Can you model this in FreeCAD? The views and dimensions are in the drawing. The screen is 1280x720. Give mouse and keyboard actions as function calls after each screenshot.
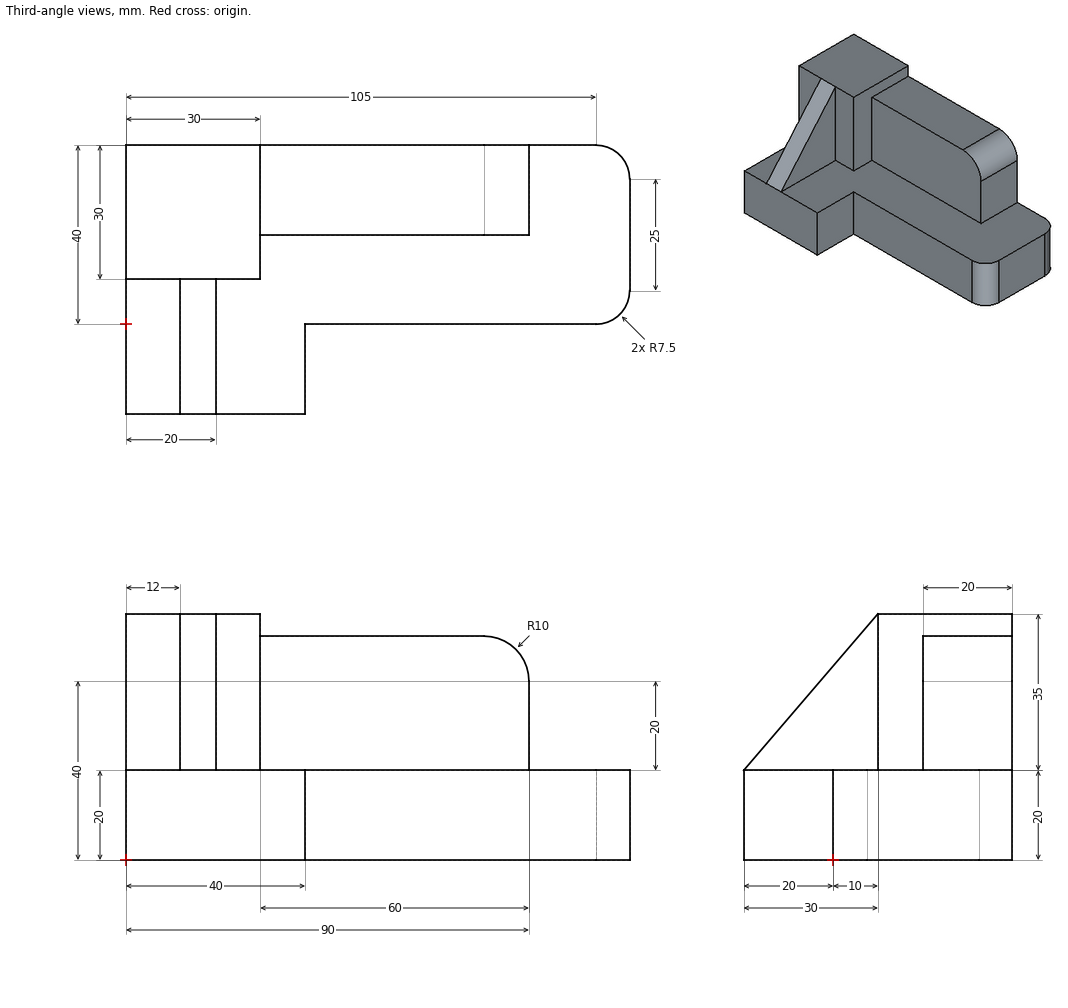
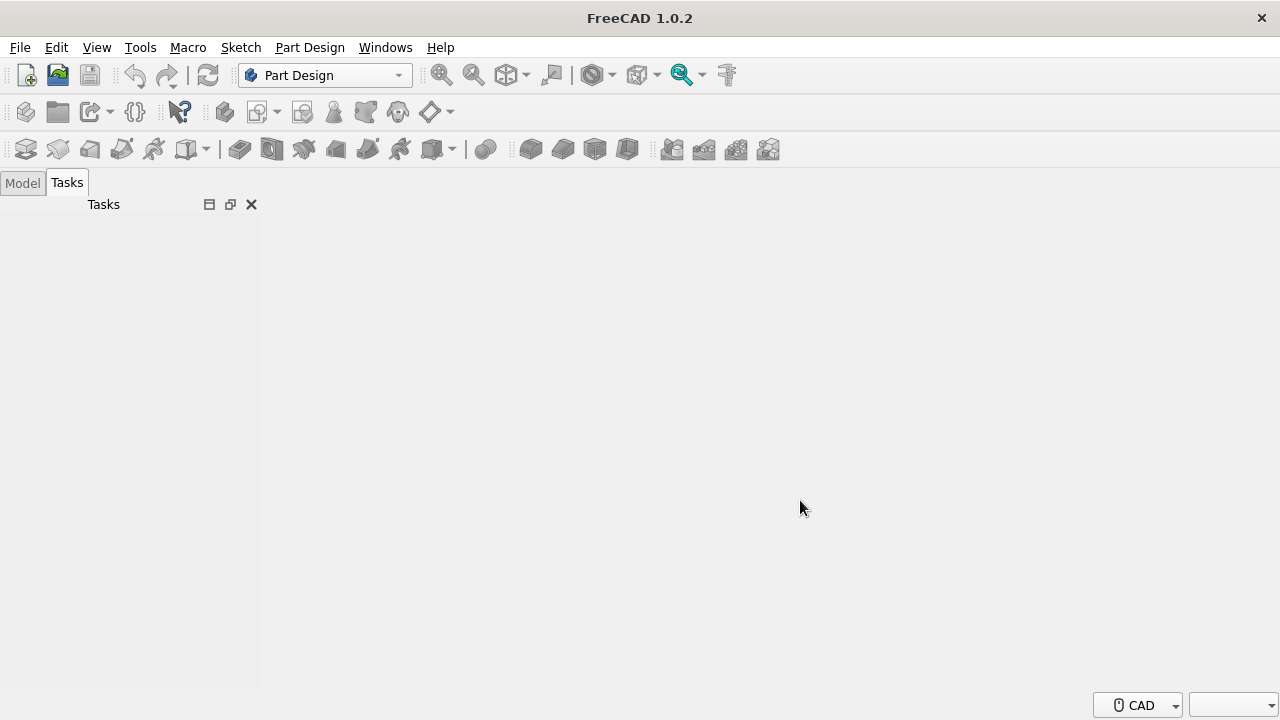
key(ctrl+n)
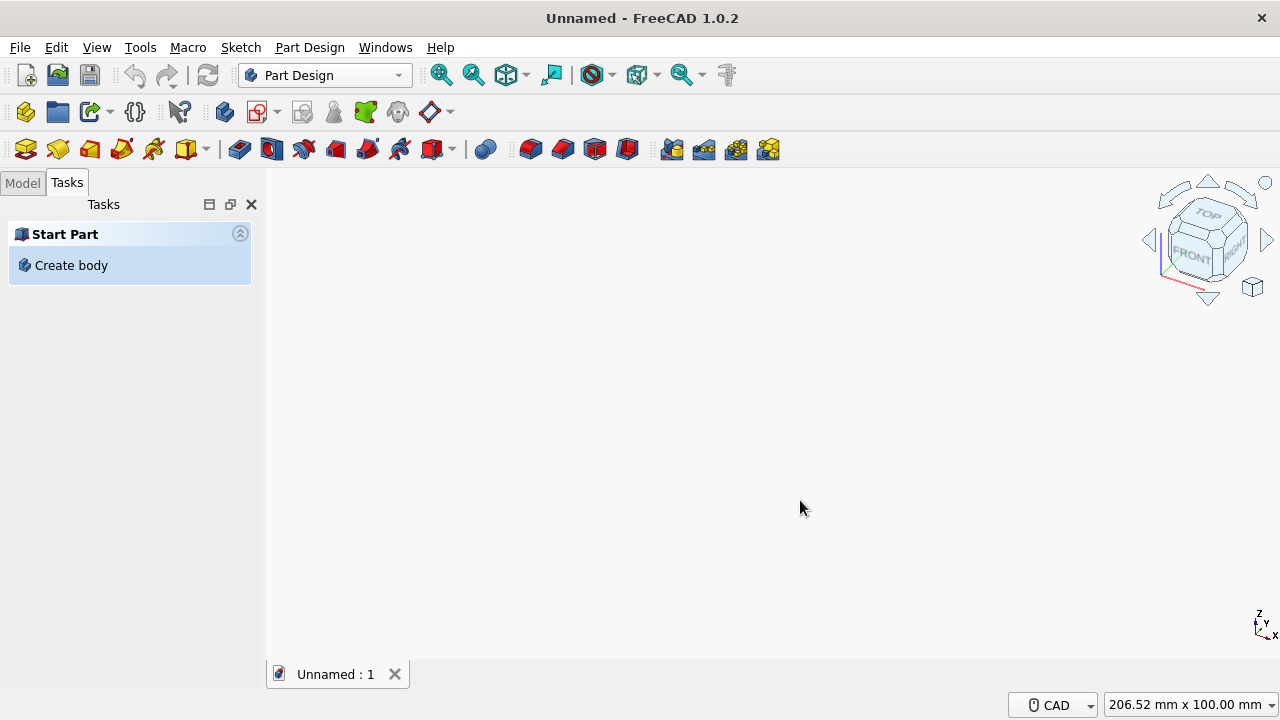
click(258, 112)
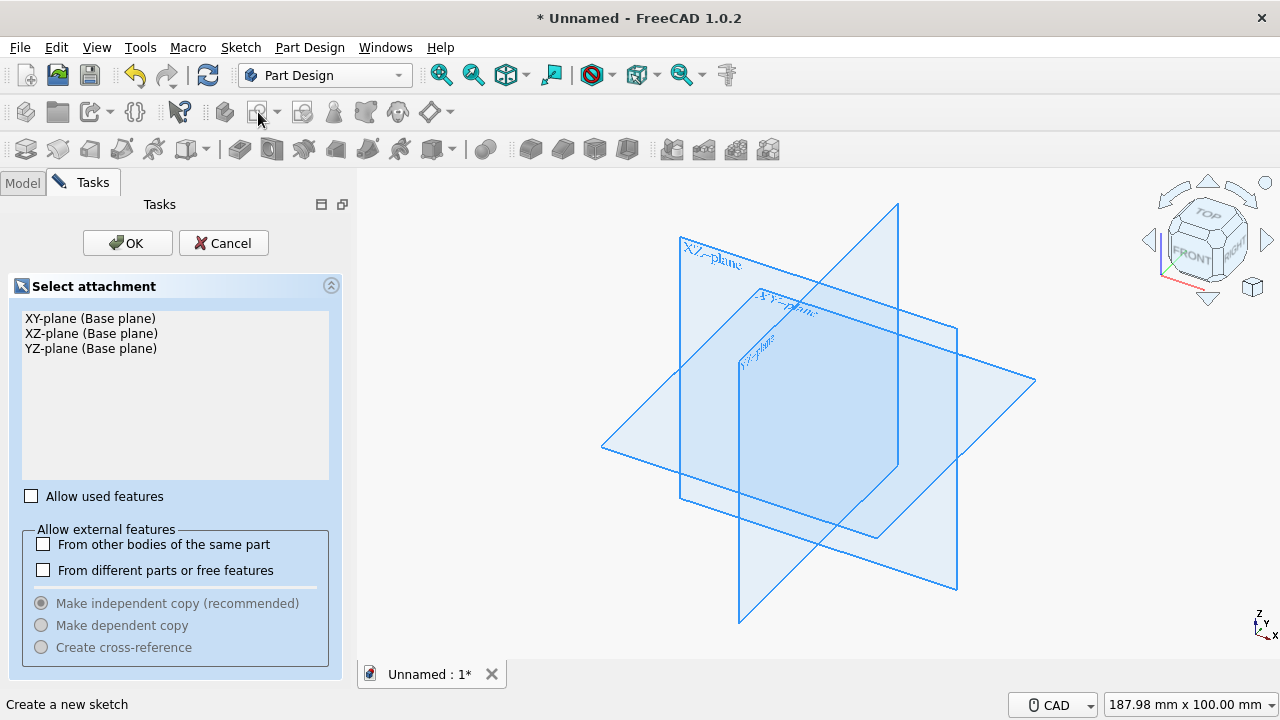
click(82, 318)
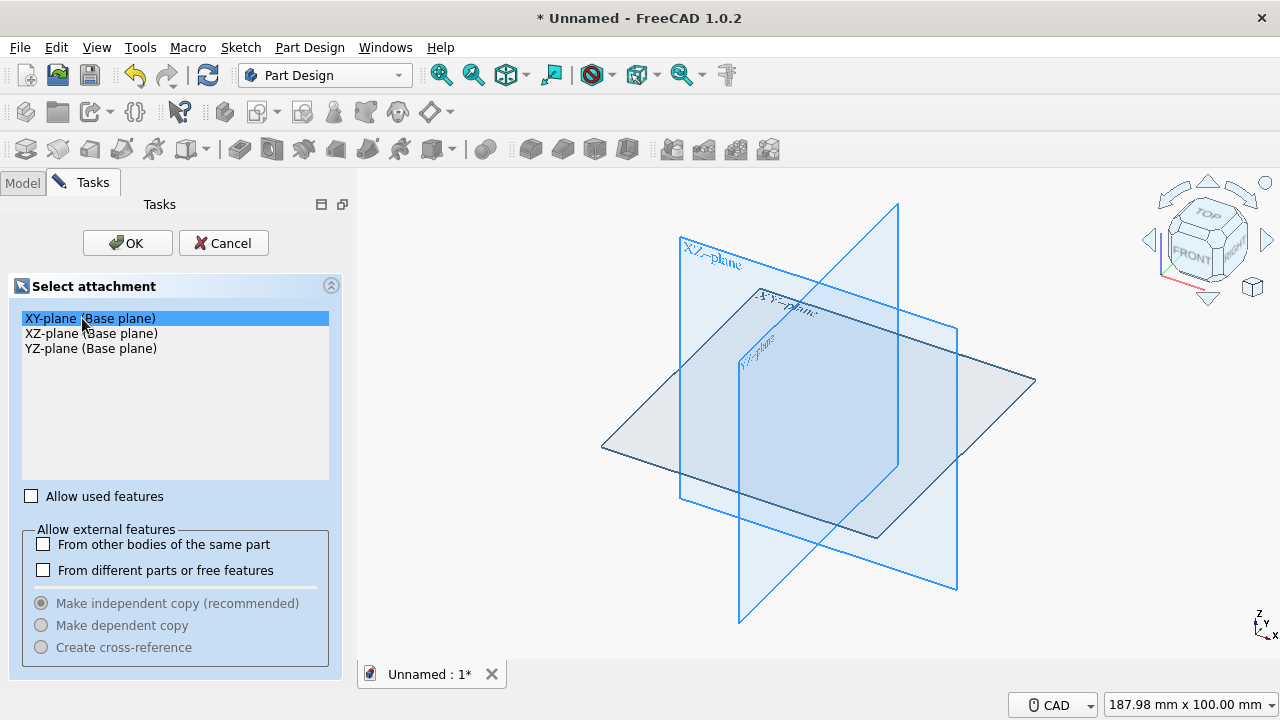
click(128, 243)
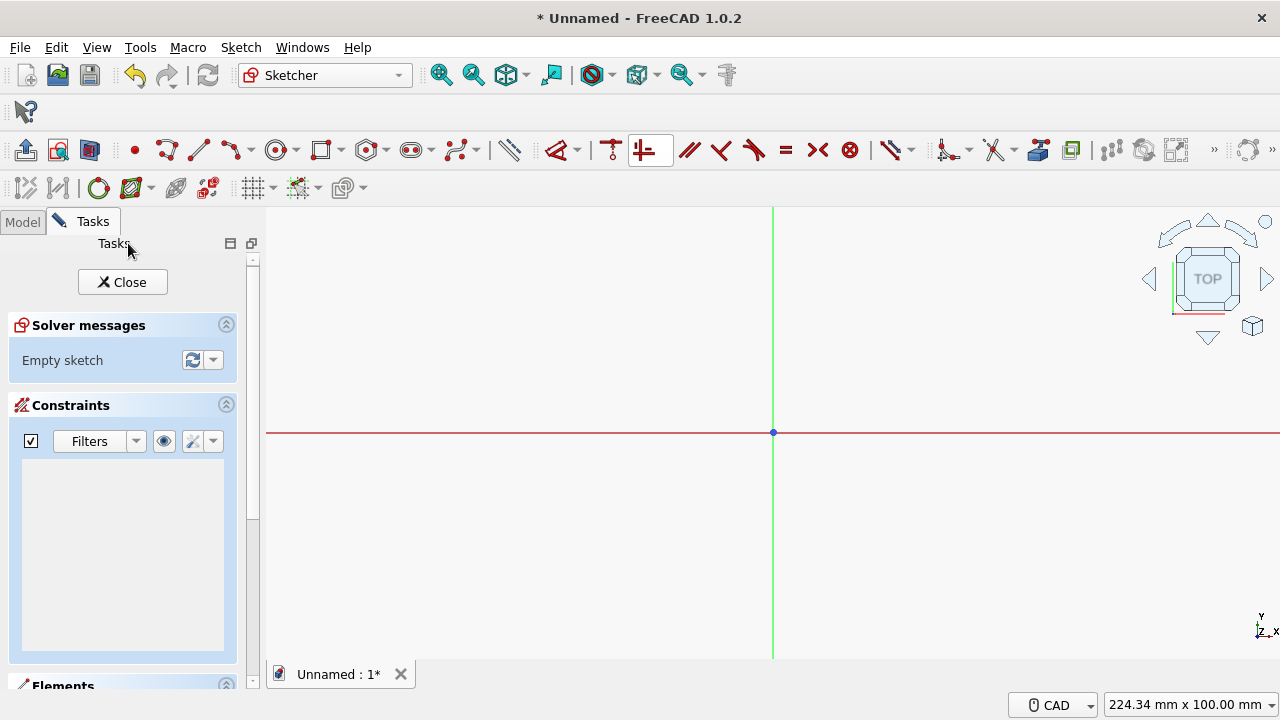
scroll(294, 617, down, 2)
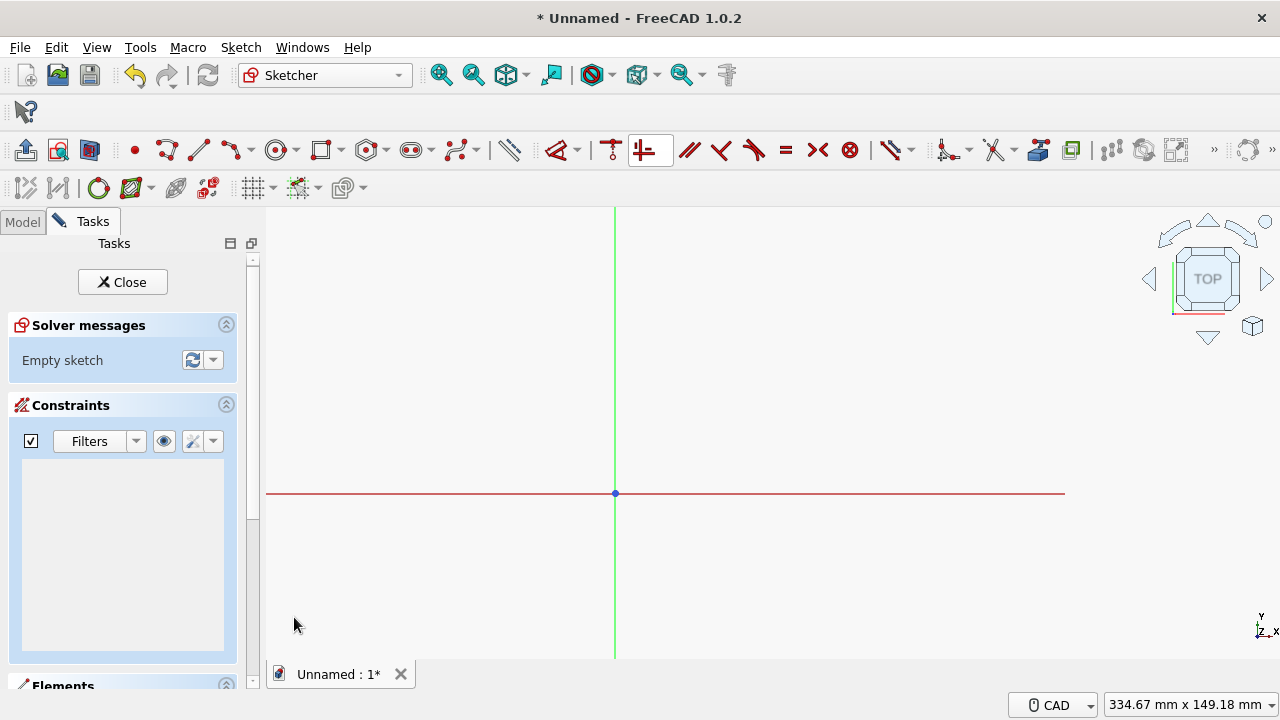
scroll(884, 434, up, 3)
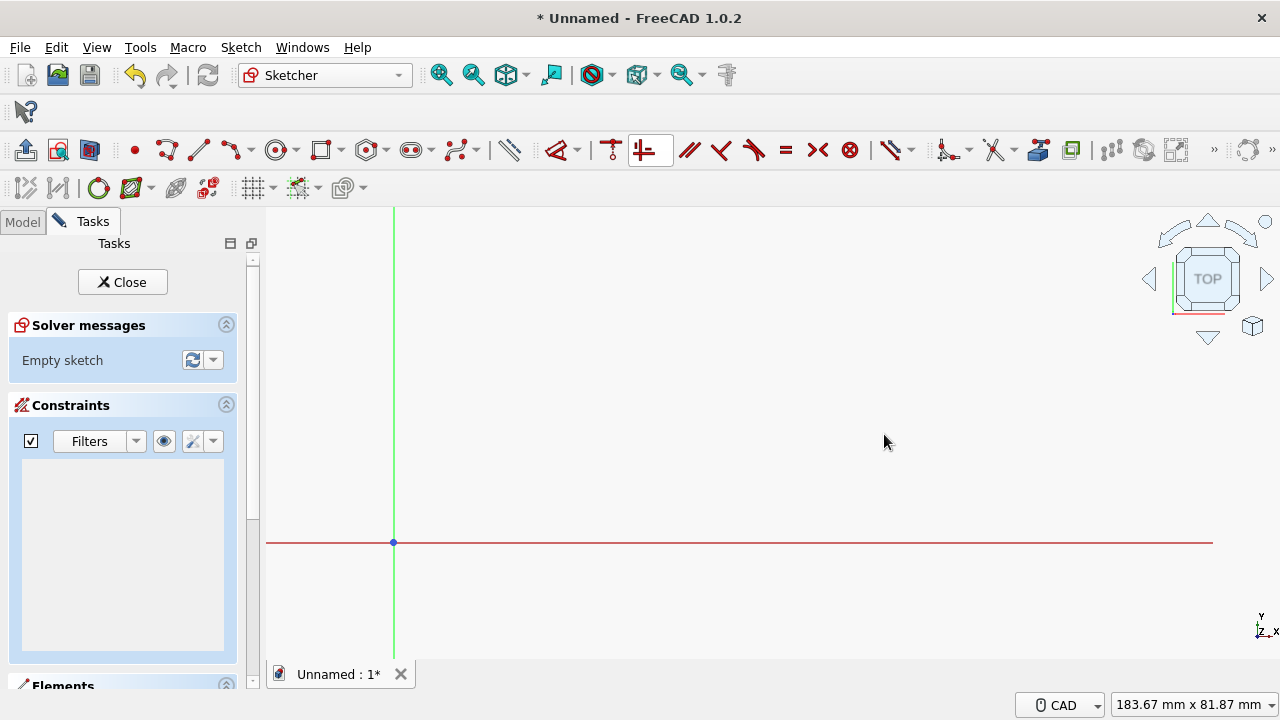
key(g)
key(l)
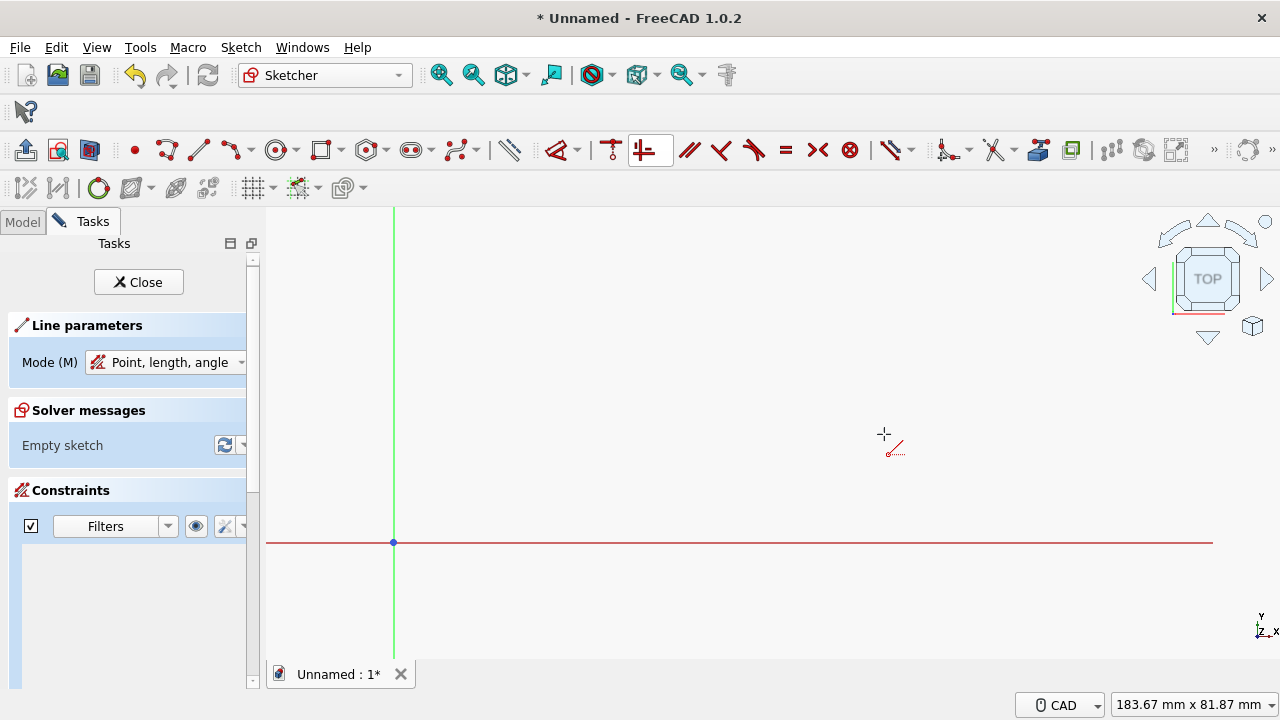
click(1015, 501)
click(1015, 363)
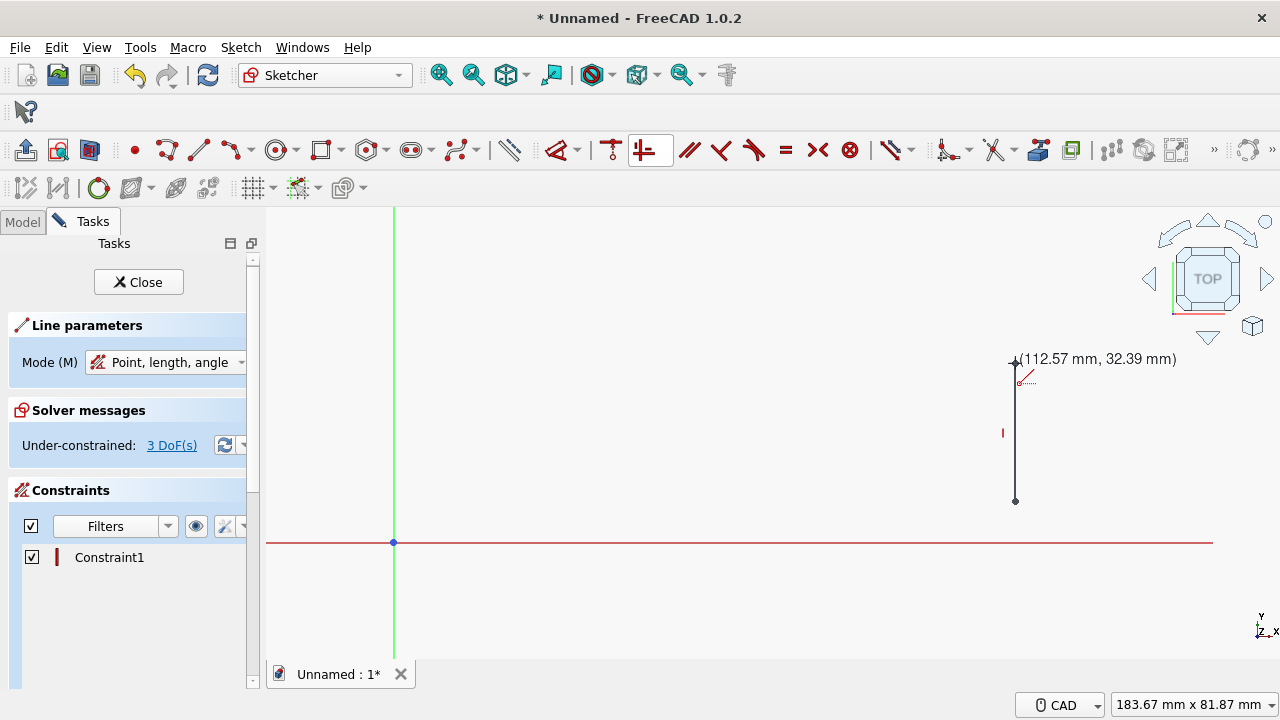
key(g)
key(m)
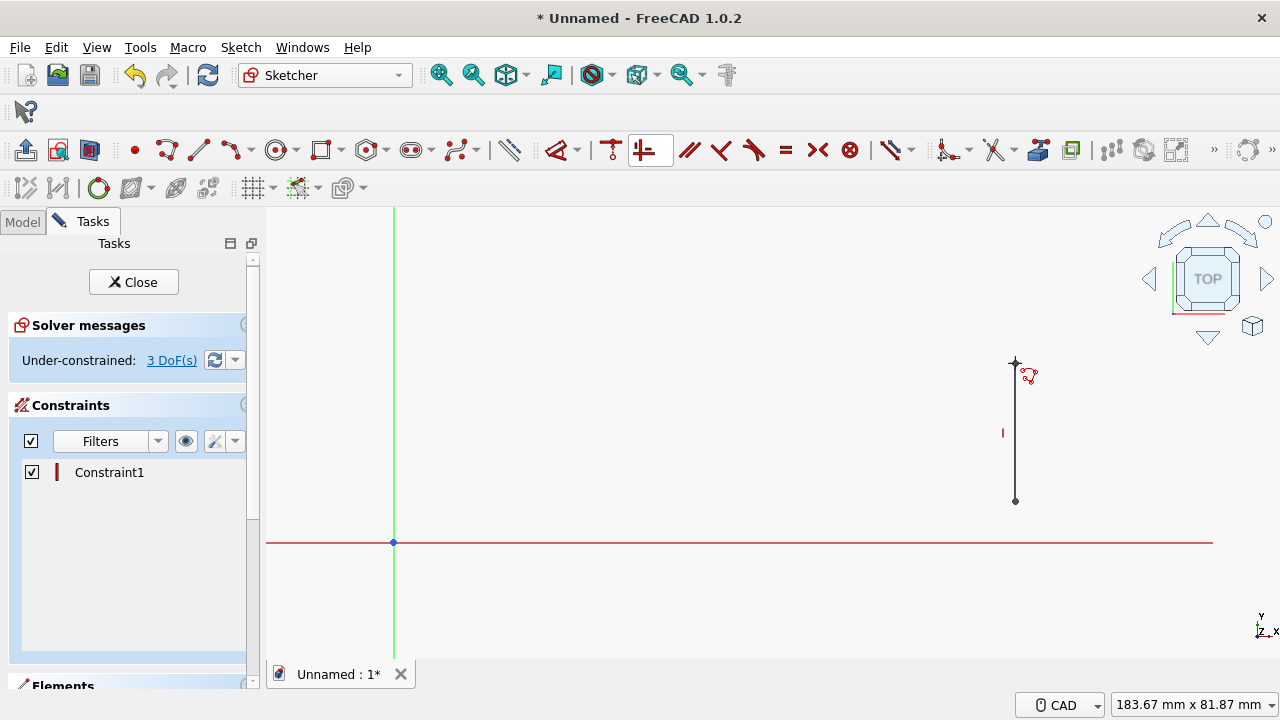
click(973, 322)
click(394, 322)
click(394, 543)
click(973, 534)
right_click(973, 534)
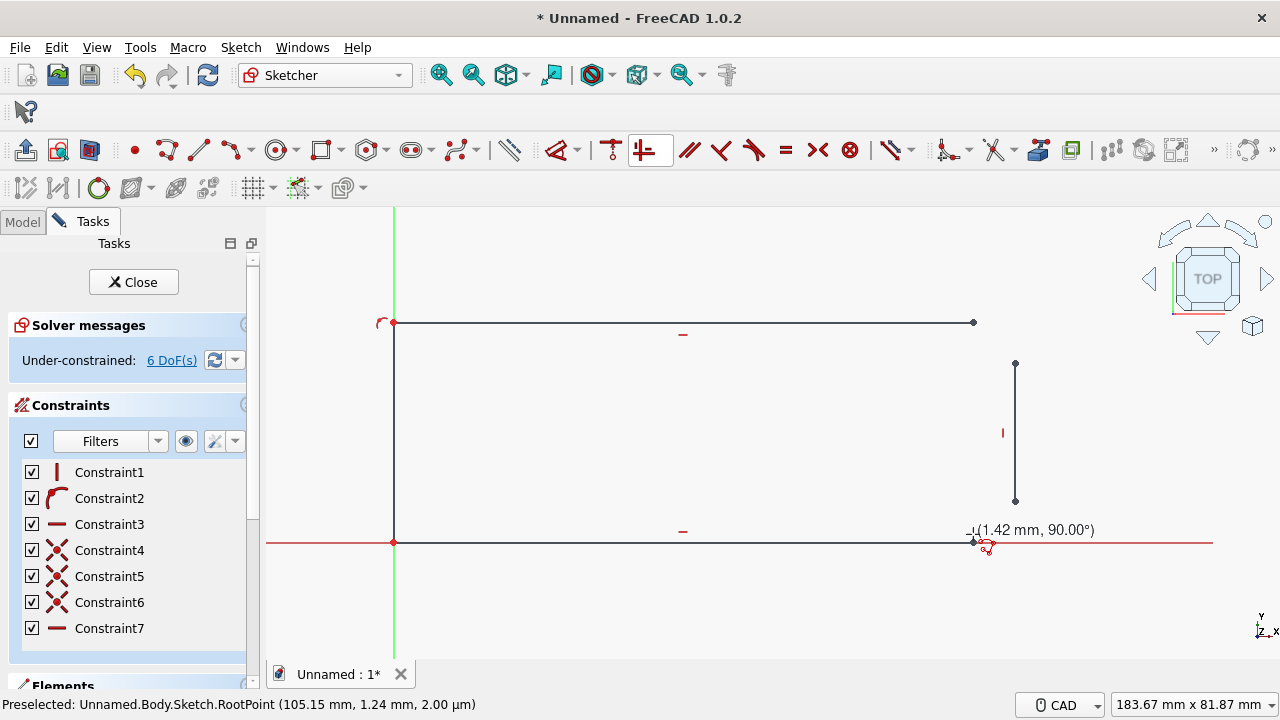
key(g)
key(3)
key(a)